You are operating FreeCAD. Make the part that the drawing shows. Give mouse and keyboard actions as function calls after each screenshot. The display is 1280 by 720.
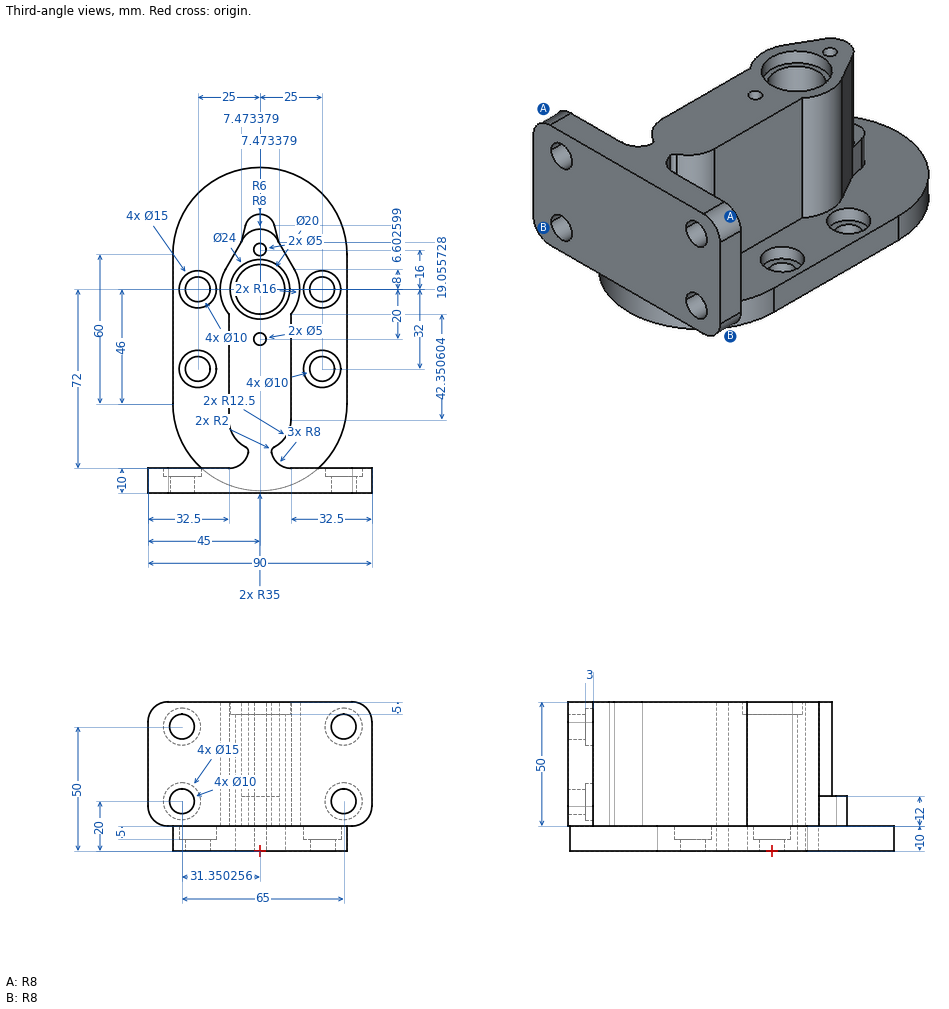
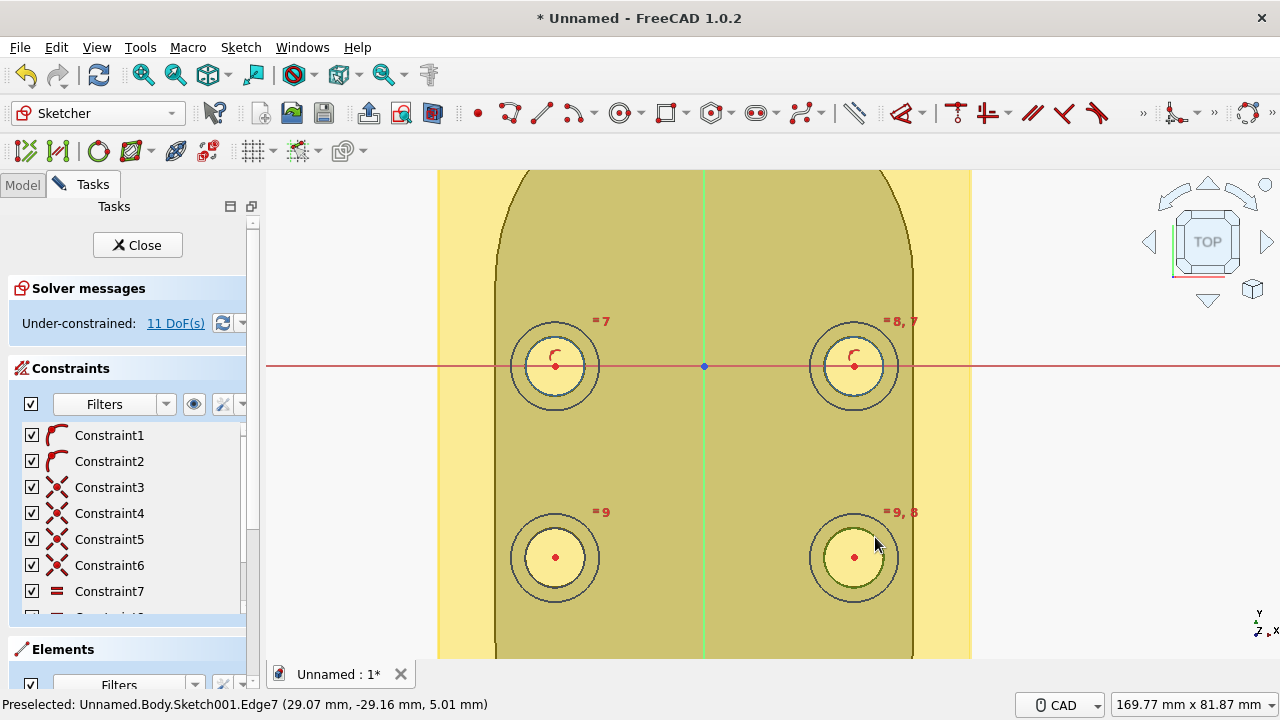
click(576, 537)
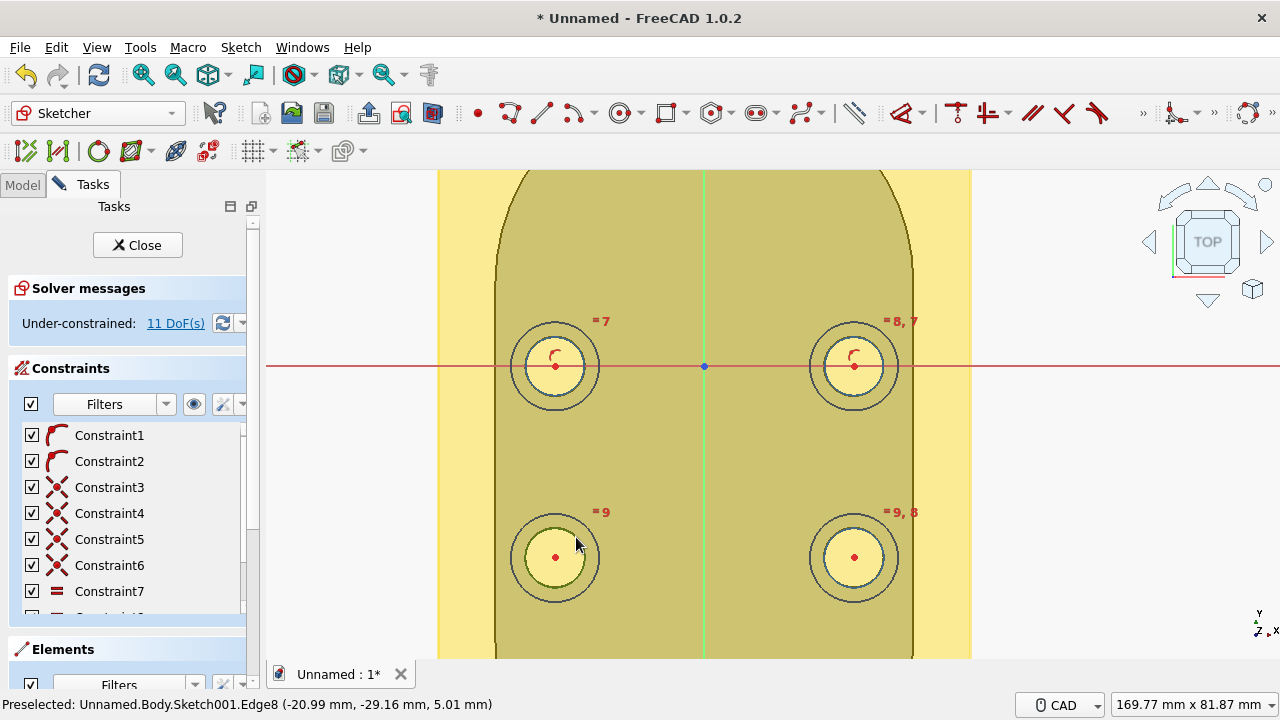
key(e)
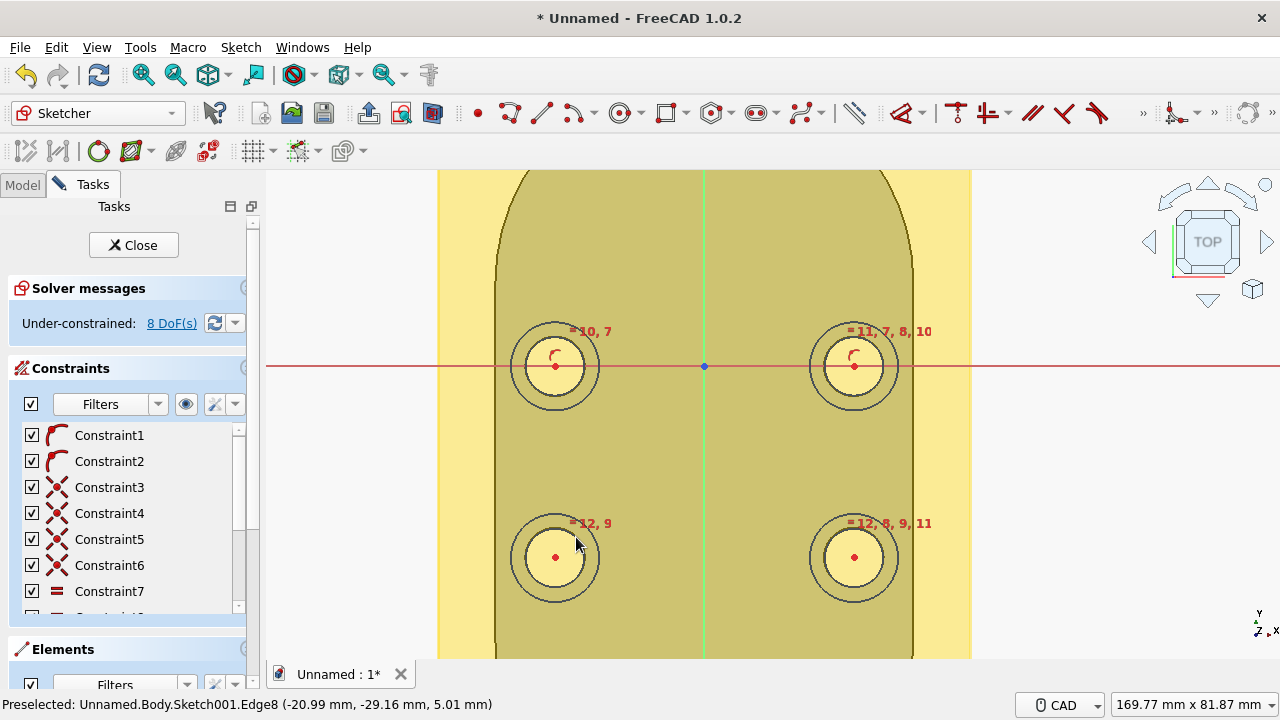
click(902, 114)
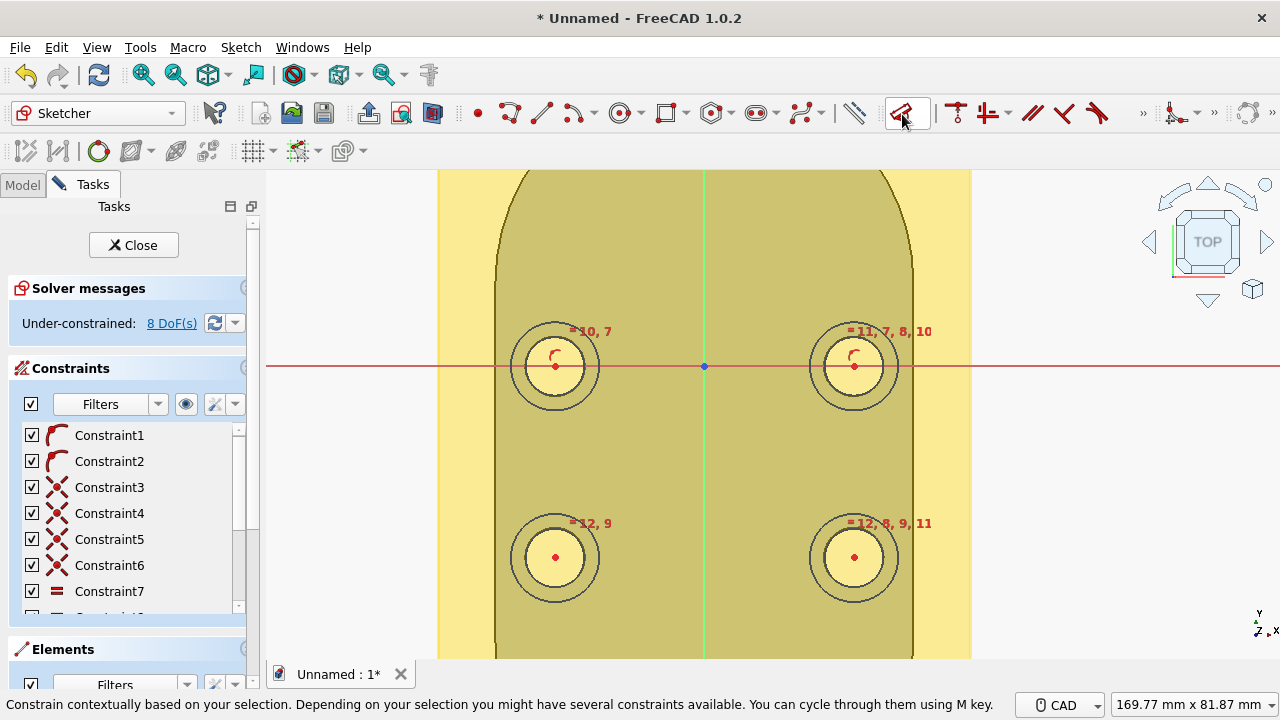
click(586, 335)
click(608, 312)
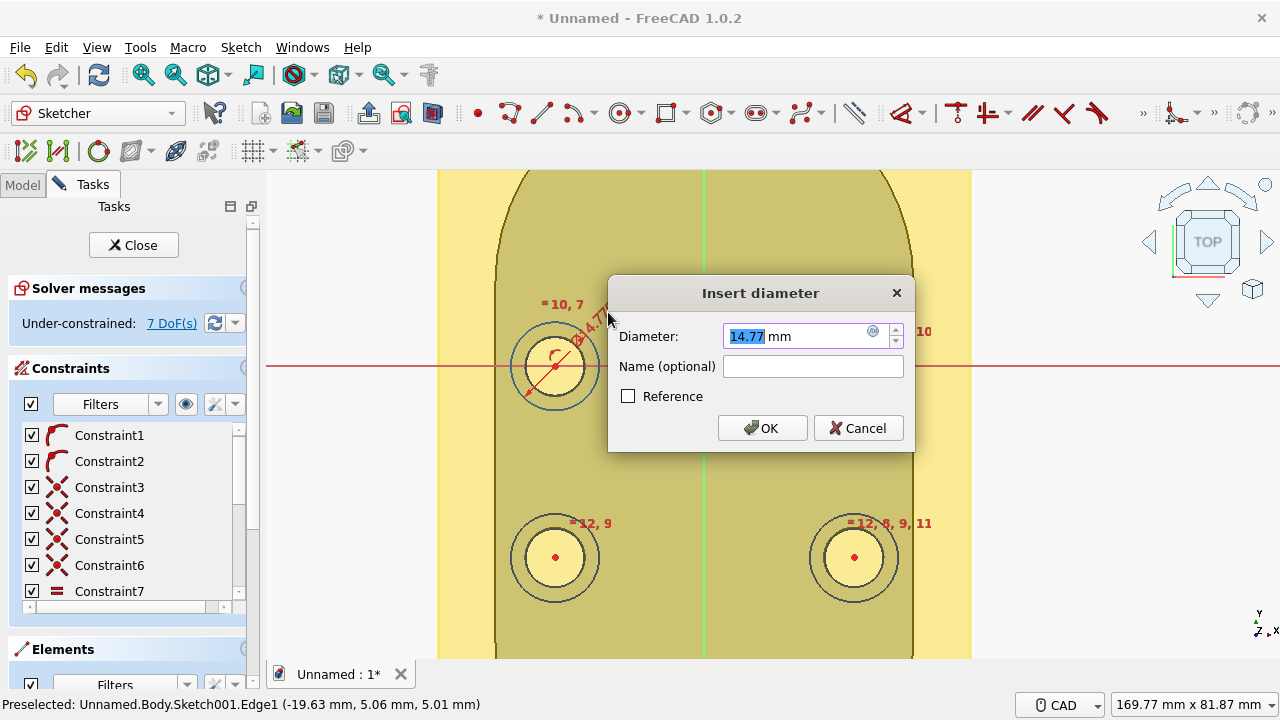
text(15)
key(Return)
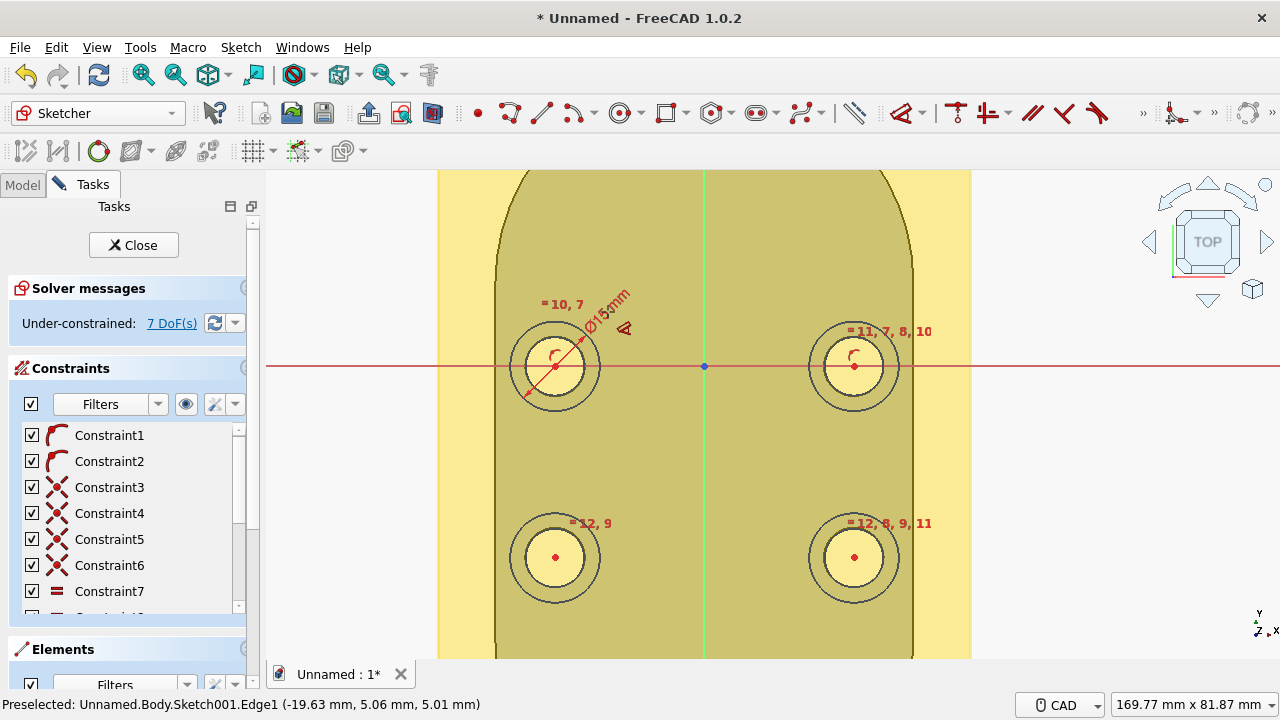
click(576, 346)
click(614, 350)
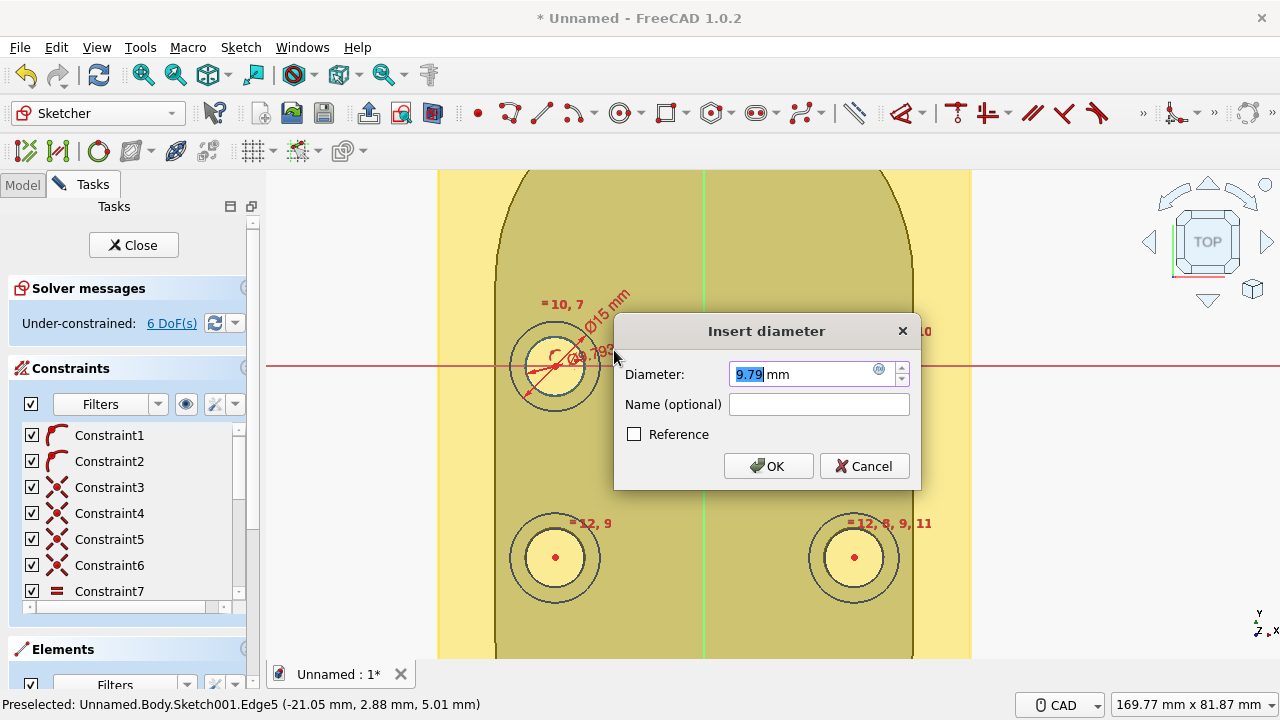
text(10)
key(Return)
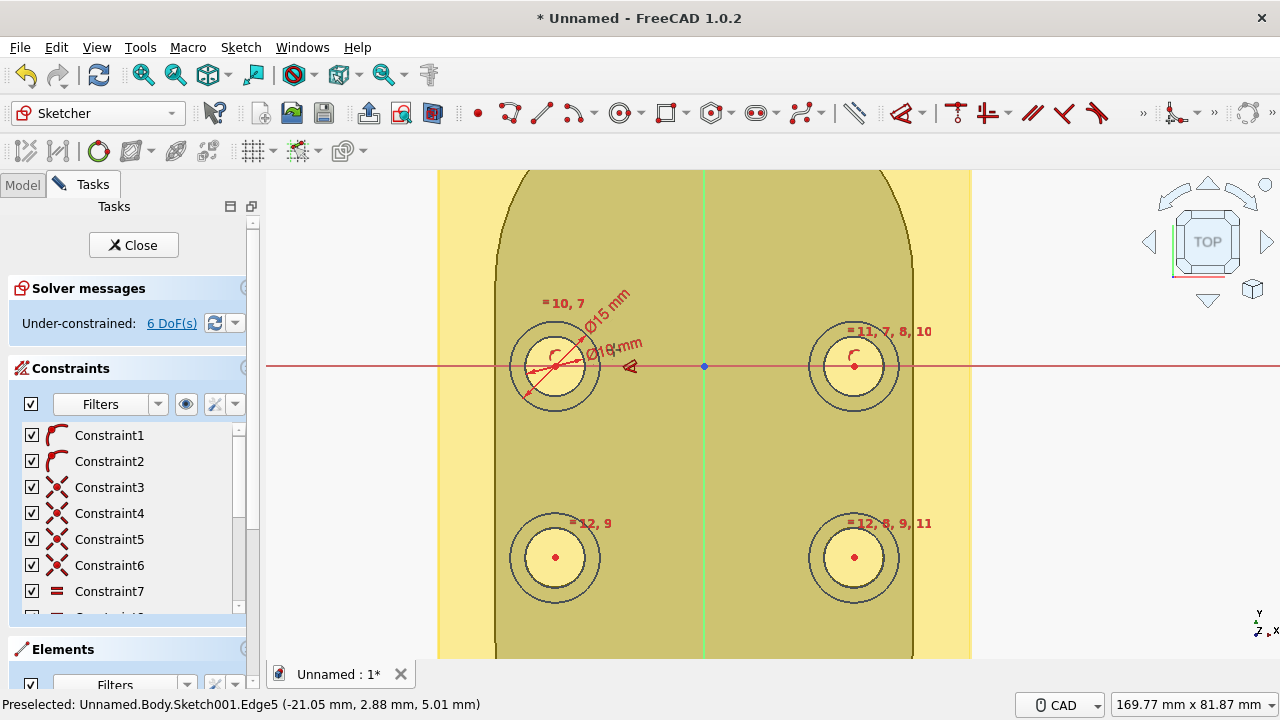
click(555, 366)
click(630, 400)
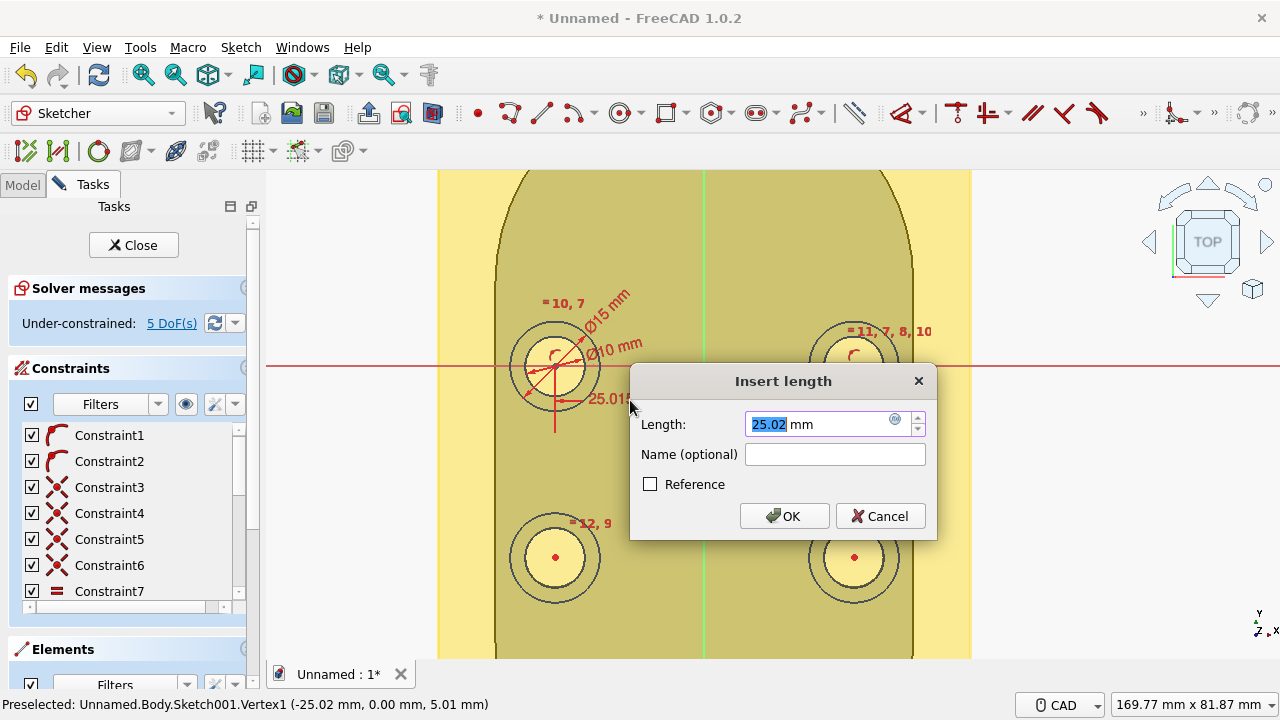
text(25)
key(Return)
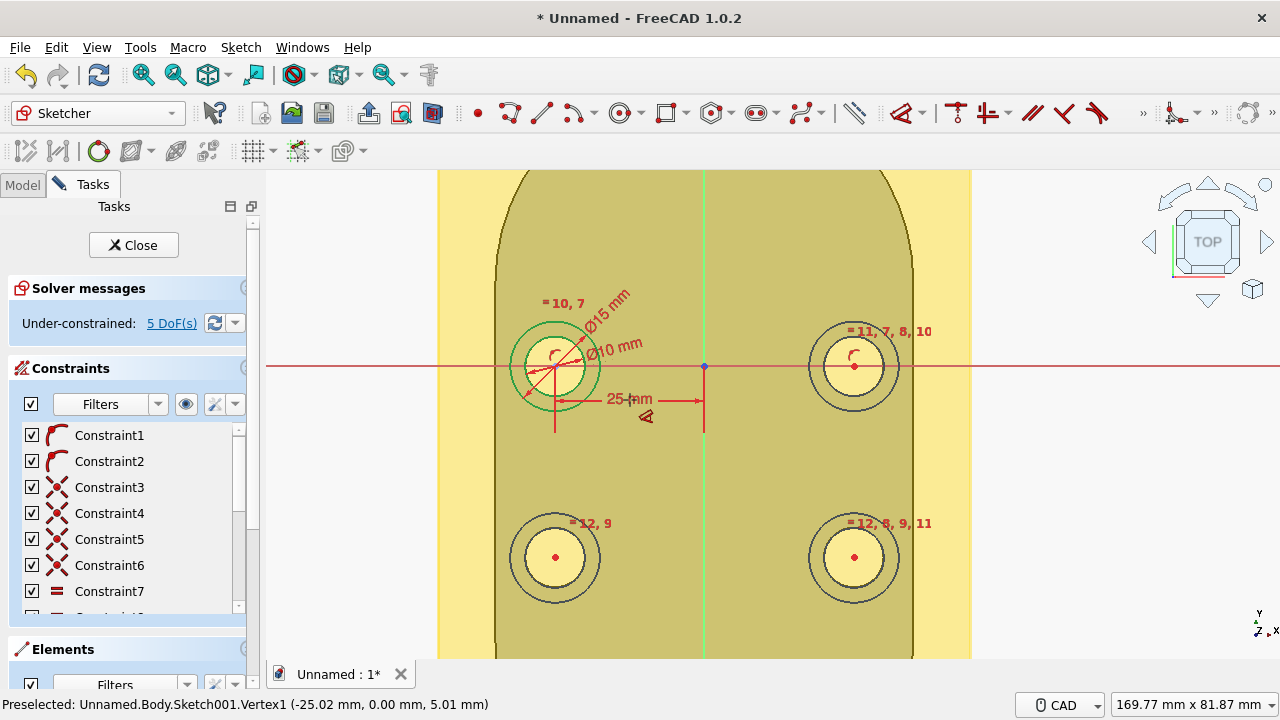
click(854, 366)
click(779, 332)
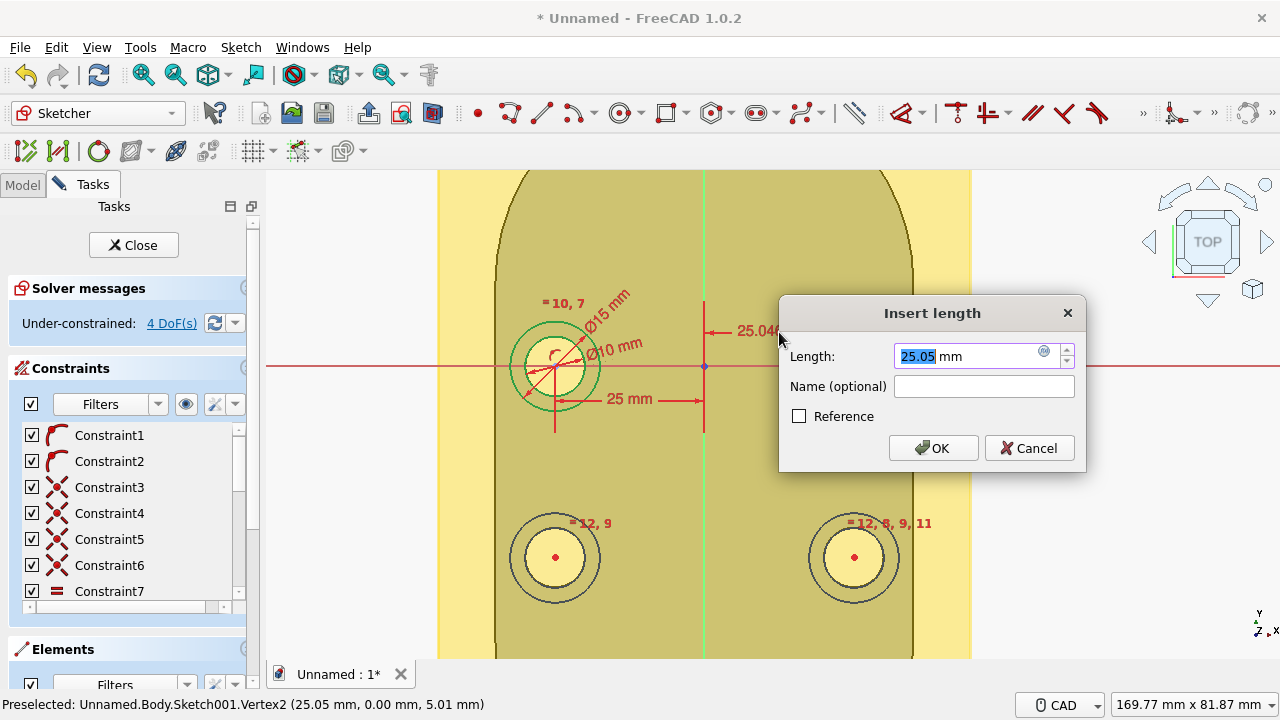
text(25)
key(Return)